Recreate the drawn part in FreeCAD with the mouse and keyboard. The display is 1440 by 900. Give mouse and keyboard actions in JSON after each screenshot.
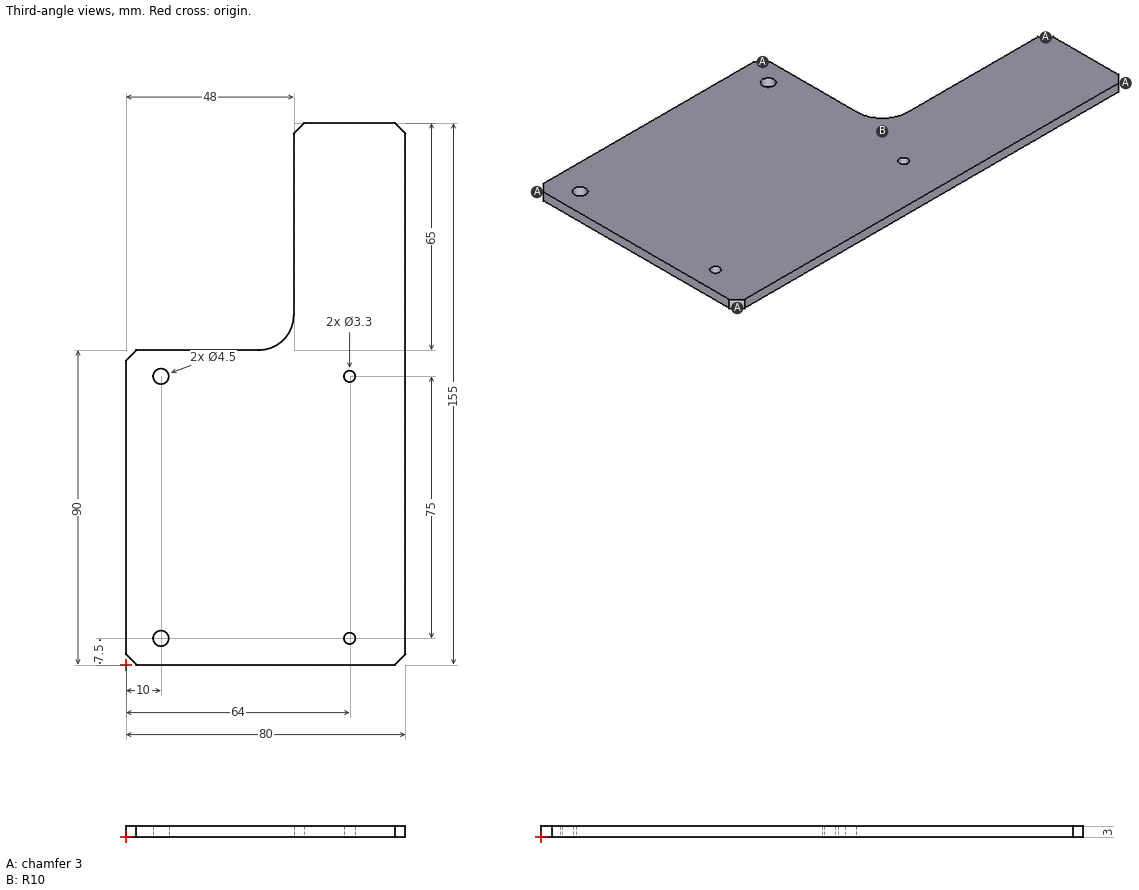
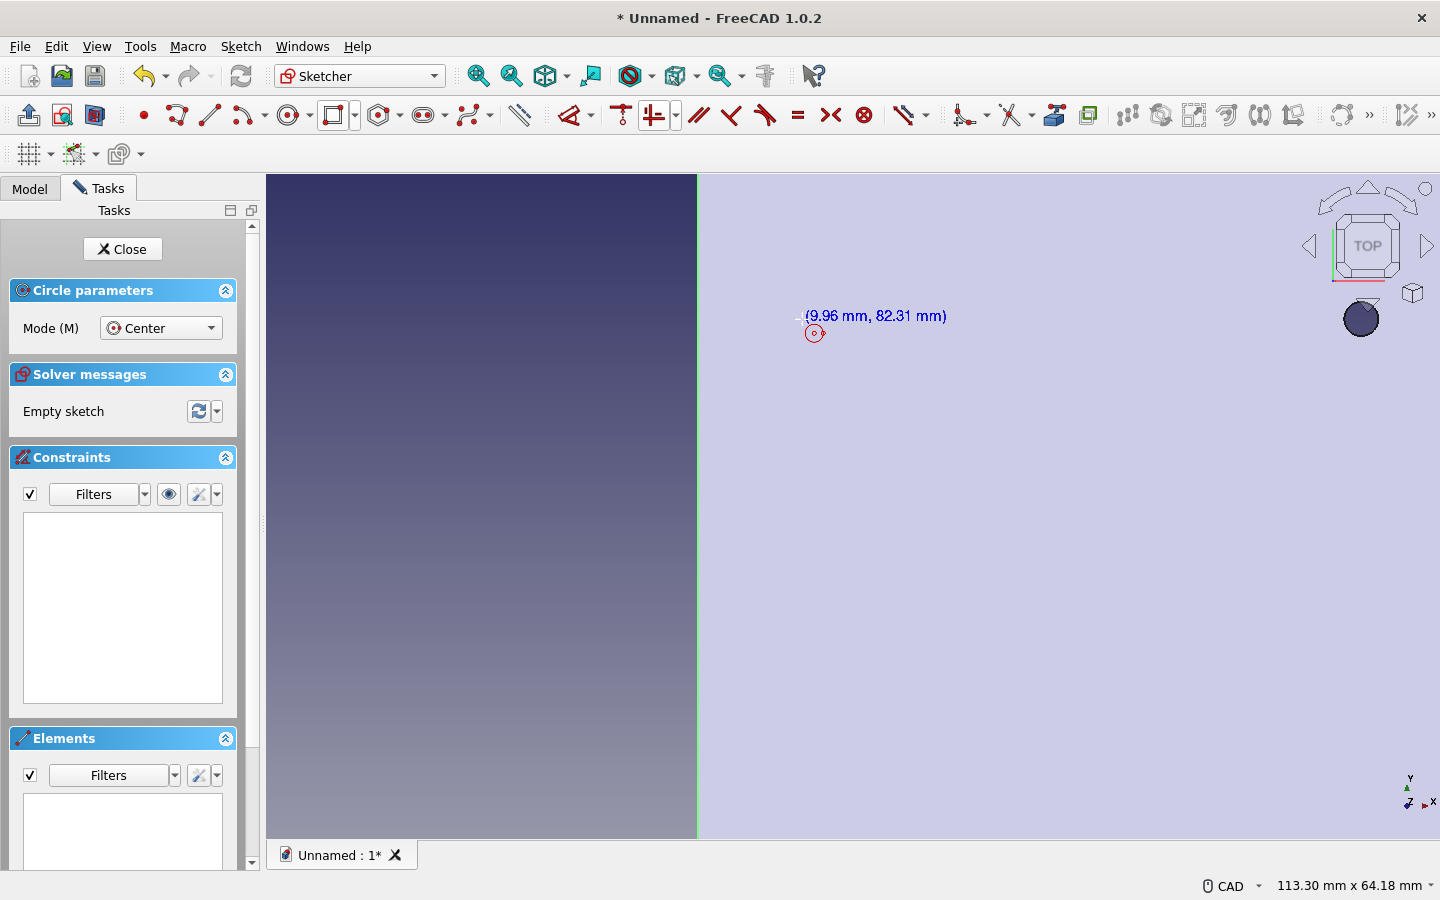
{"action": "left_click", "coordinate": [802, 319]}
{"action": "mouse_move", "coordinate": [818, 303]}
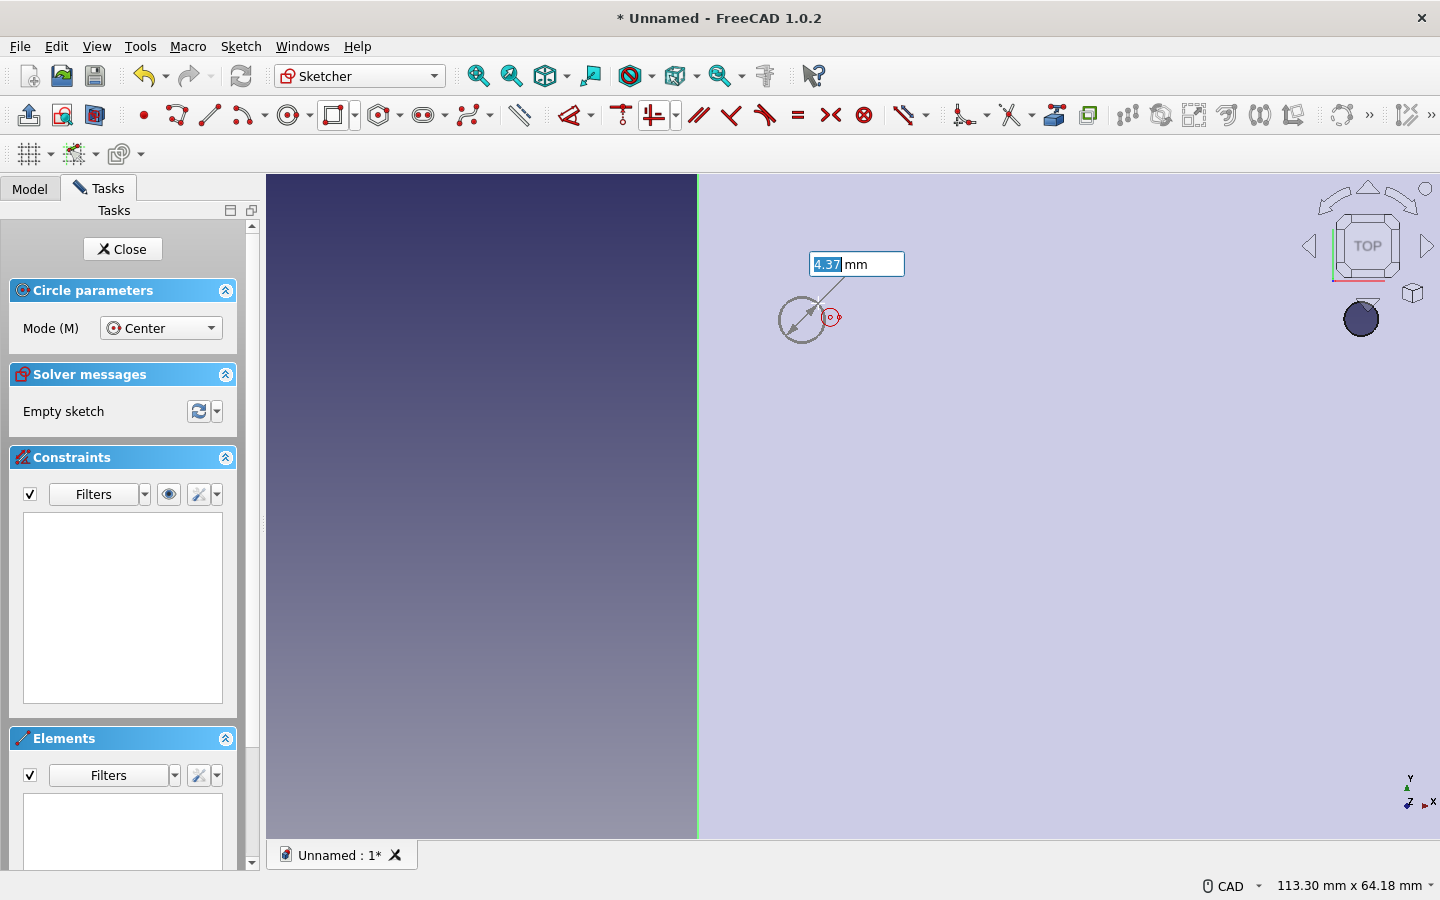
{"action": "type", "text": "4.5"}
{"action": "key", "text": "Return"}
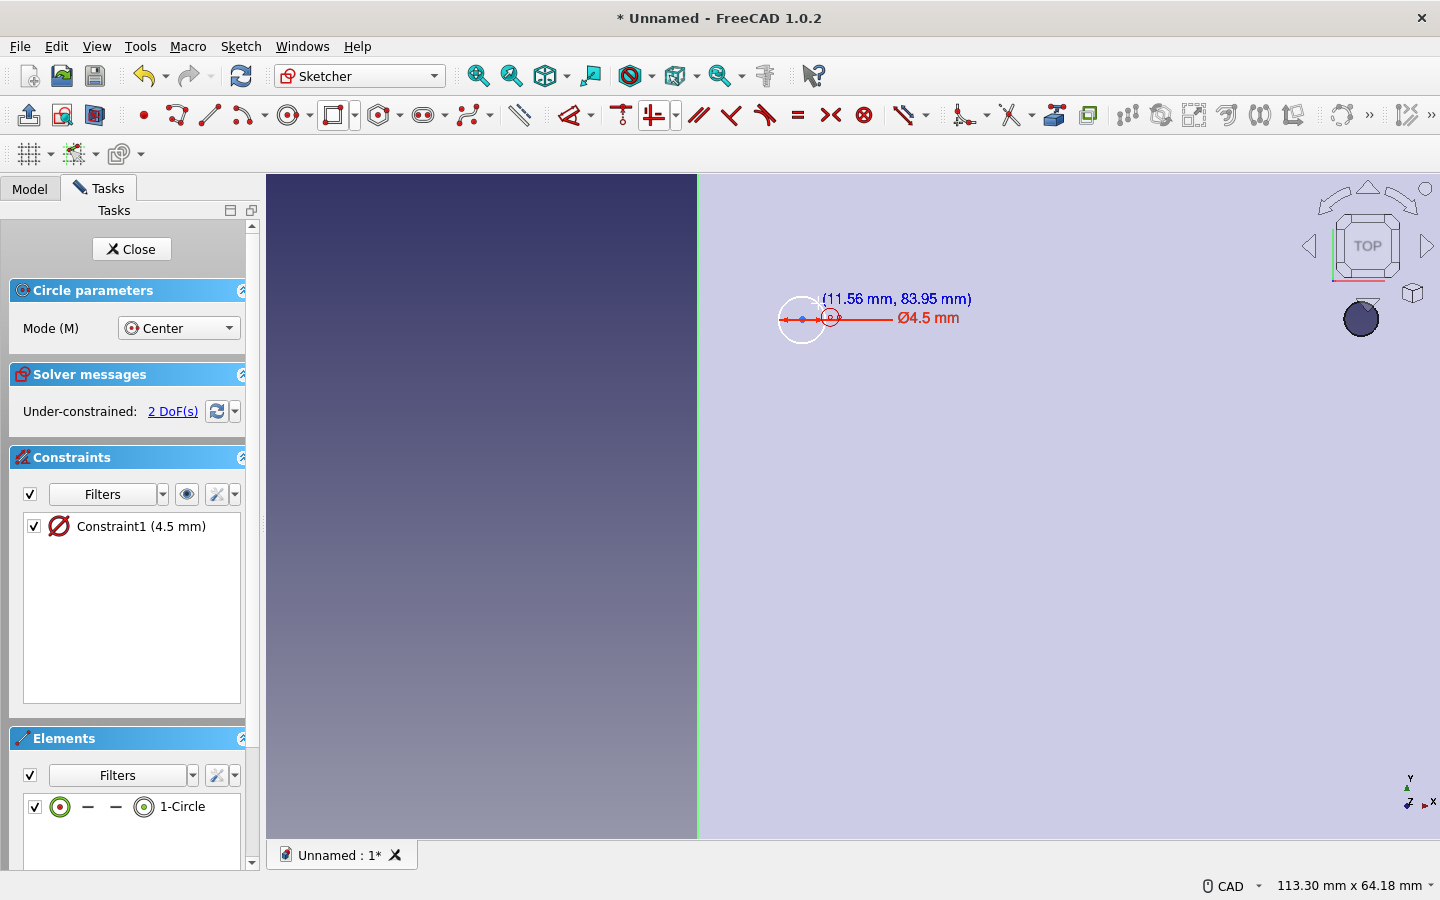
{"action": "scroll", "coordinate": [803, 320], "scroll_direction": "down", "scroll_amount": 4}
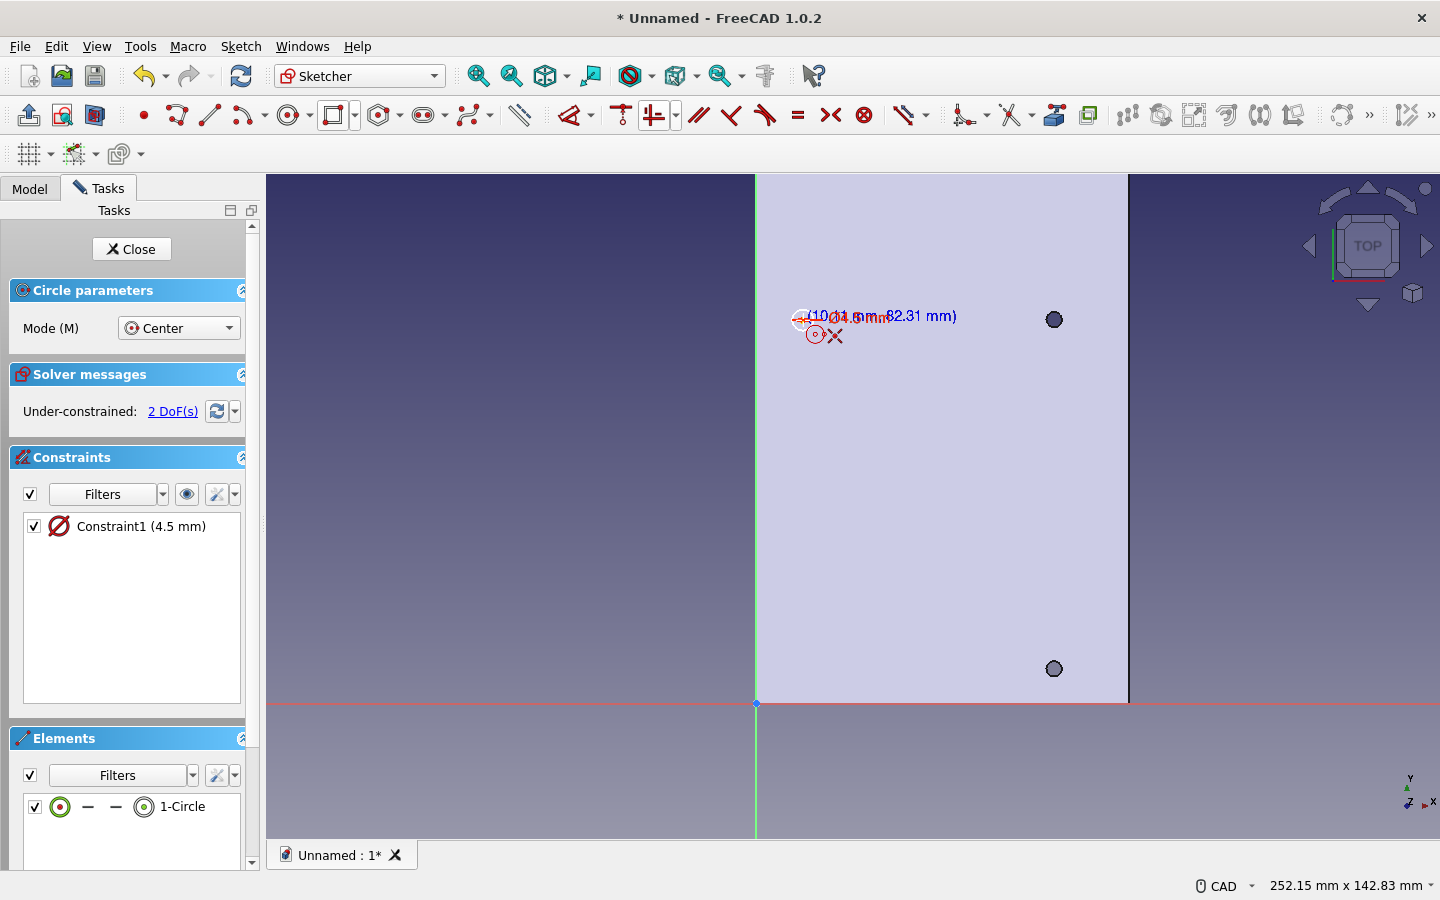
{"action": "scroll", "coordinate": [803, 669], "scroll_direction": "up", "scroll_amount": 4}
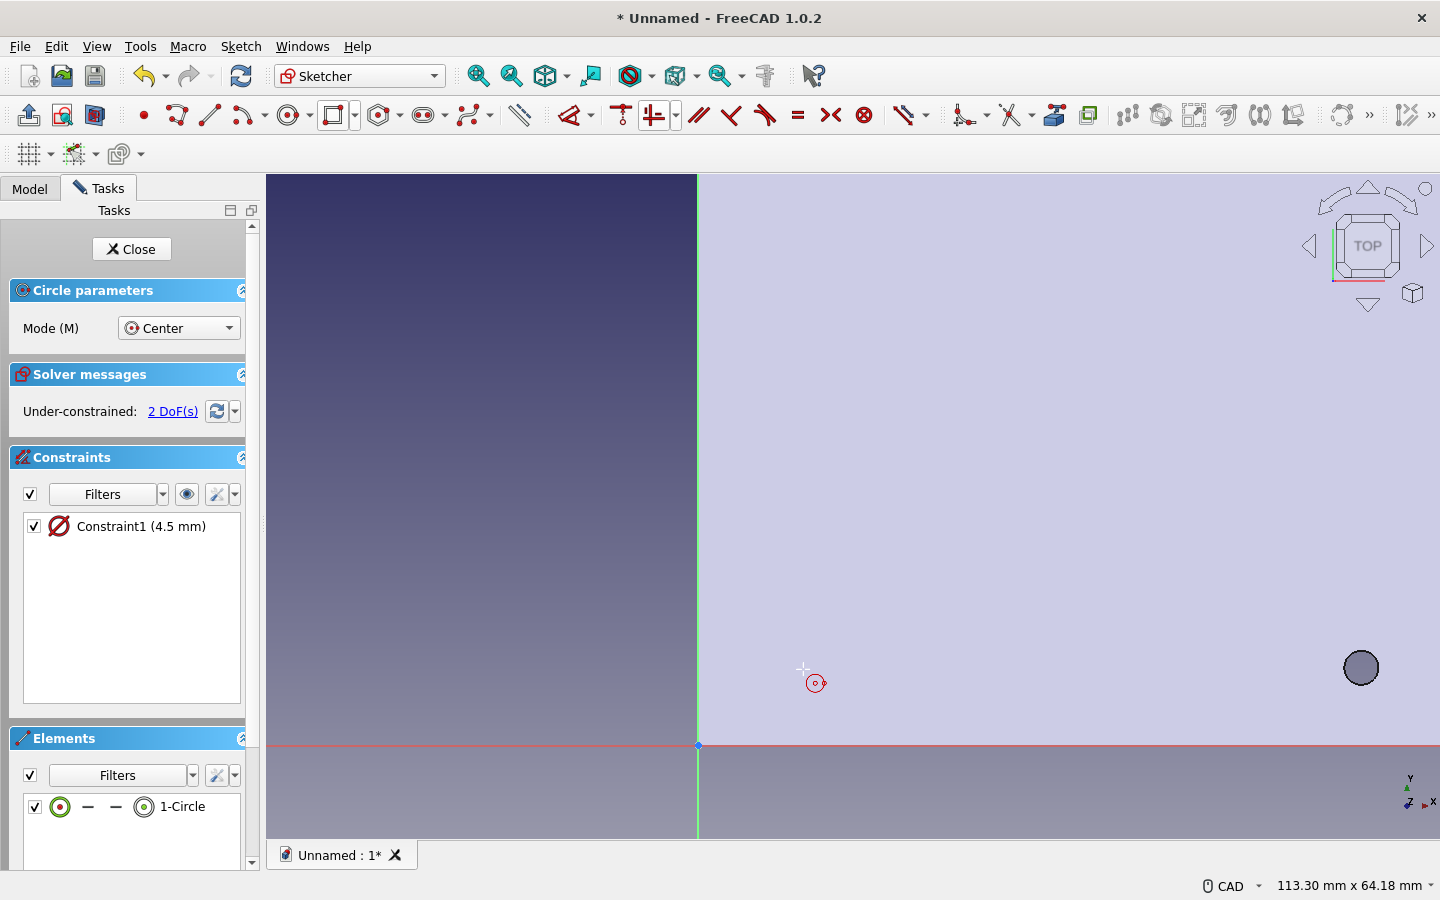
{"action": "left_click", "coordinate": [802, 668]}
{"action": "mouse_move", "coordinate": [818, 651]}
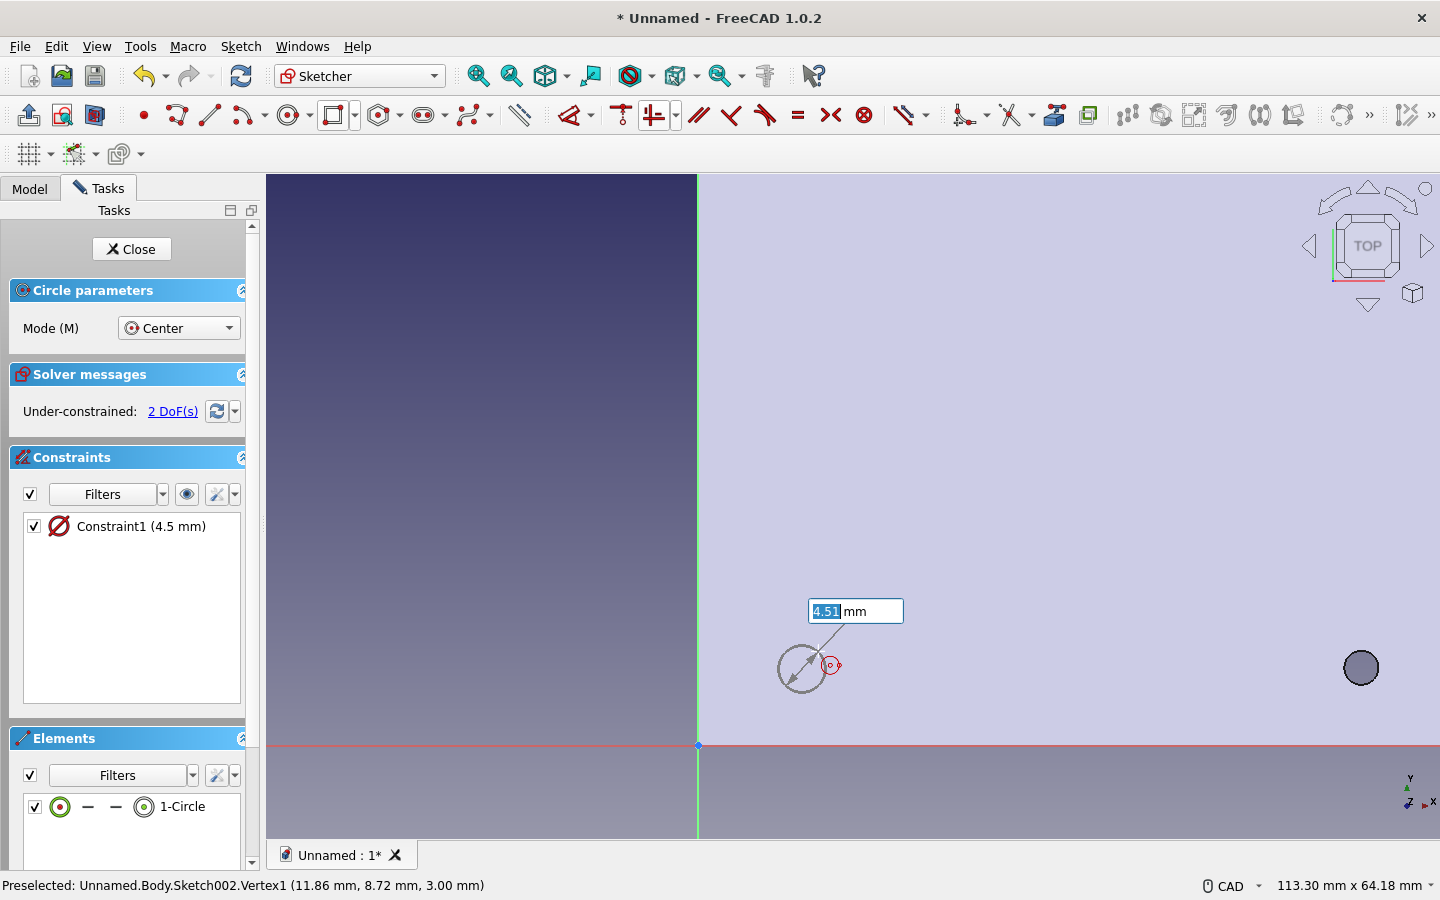
{"action": "type", "text": "4.5"}
{"action": "key", "text": "Return"}
{"action": "key", "text": "Escape"}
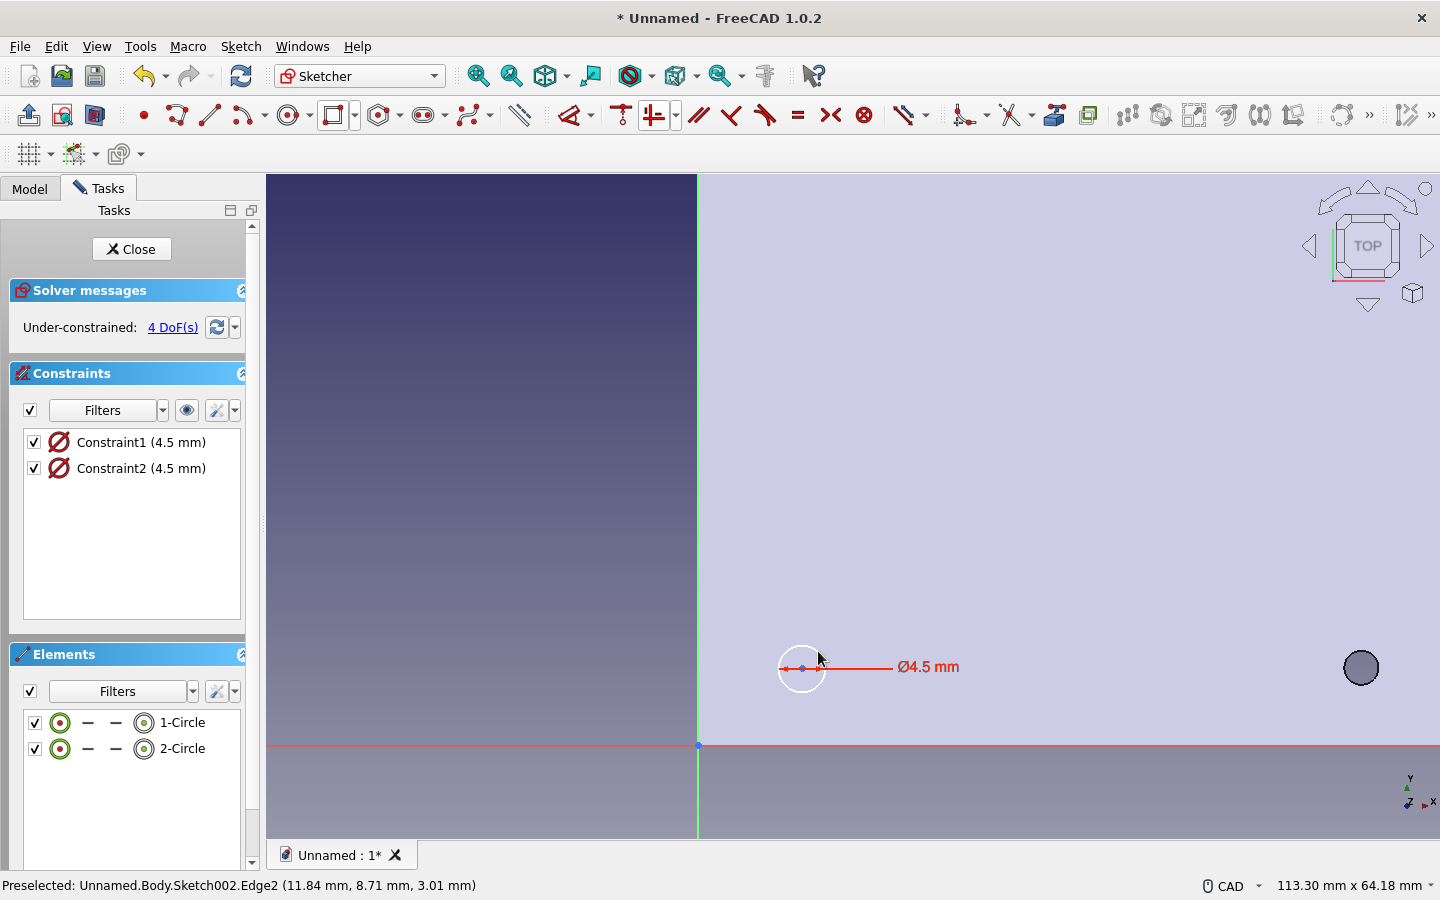
{"action": "scroll", "coordinate": [803, 670], "scroll_direction": "down", "scroll_amount": 4}